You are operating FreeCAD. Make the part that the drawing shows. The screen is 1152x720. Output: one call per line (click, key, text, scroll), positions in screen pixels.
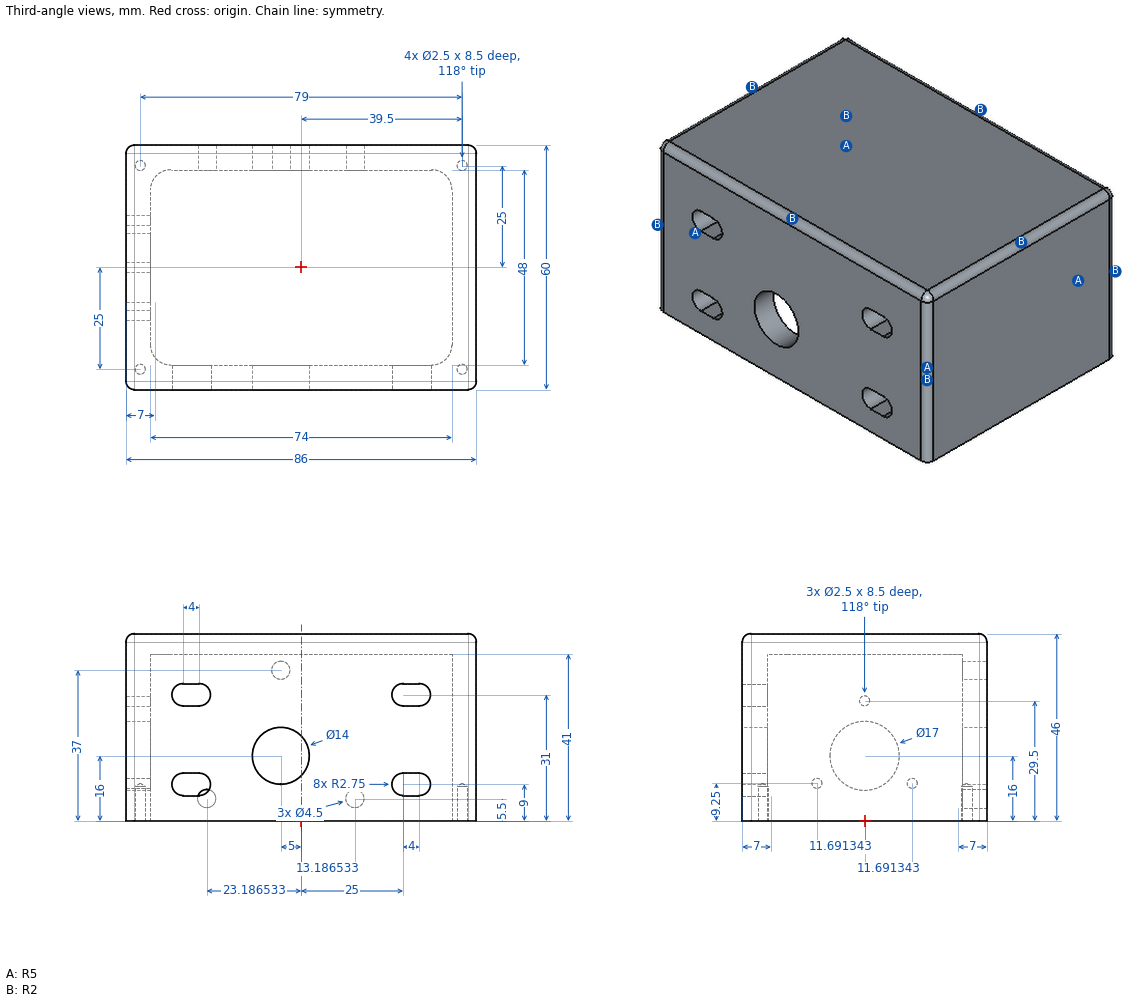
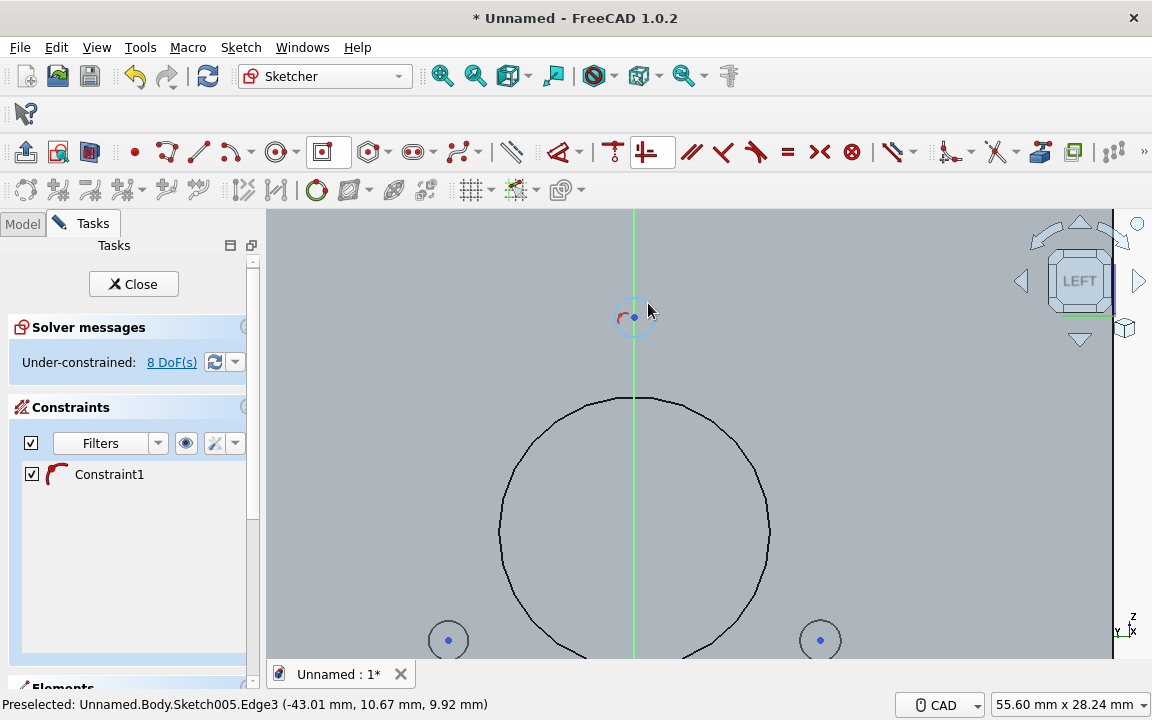
click(648, 304)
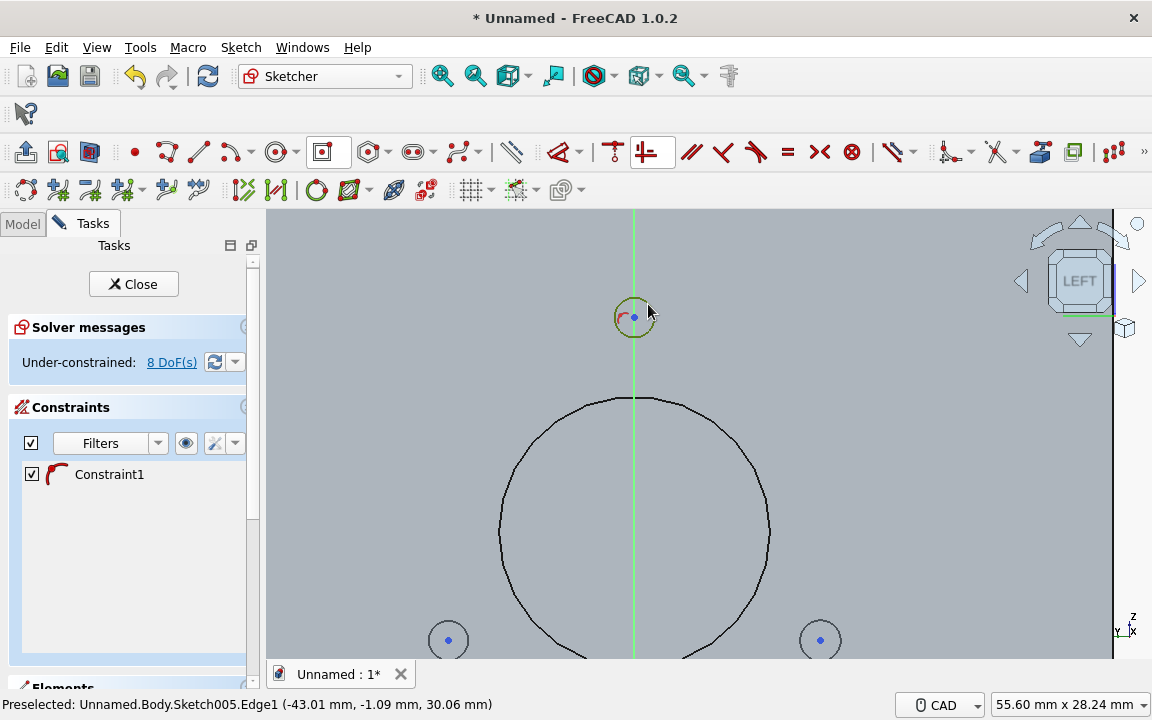
click(835, 626)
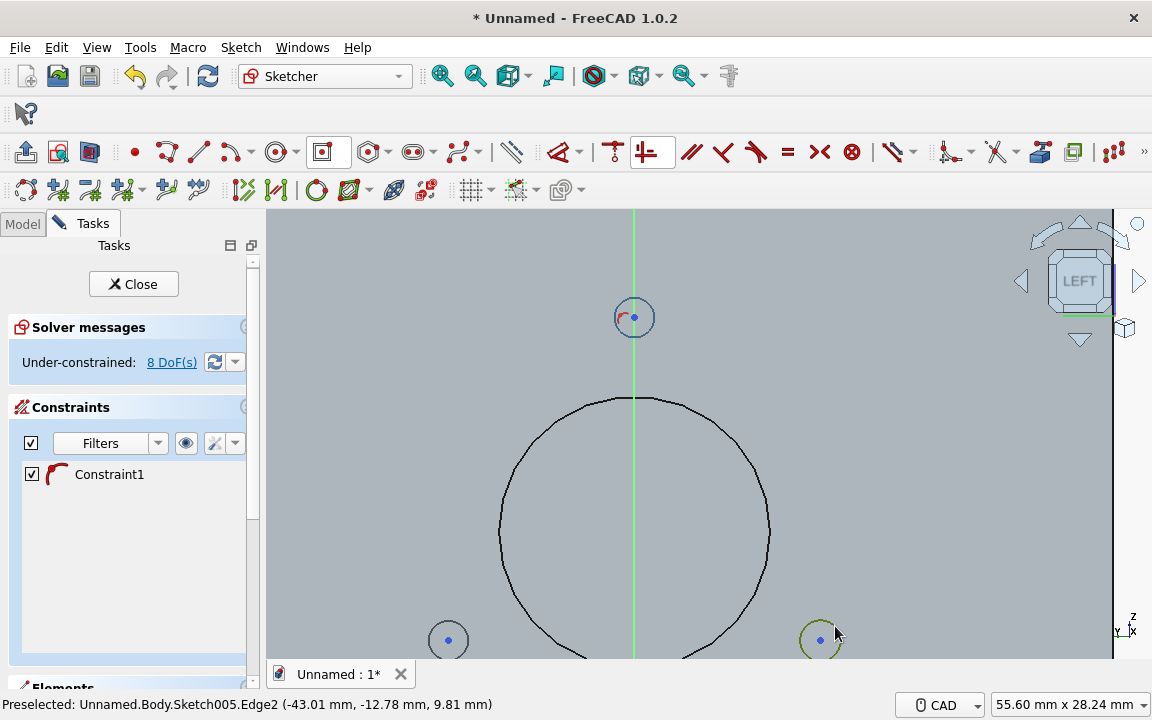
click(462, 627)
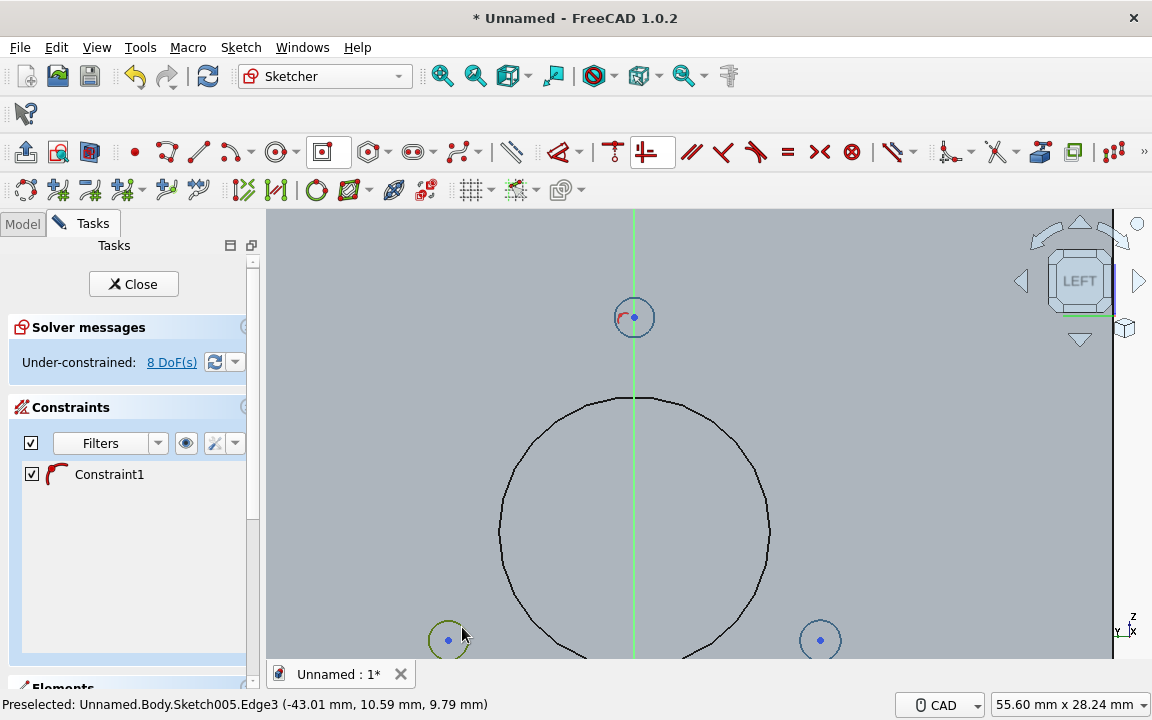
key(e)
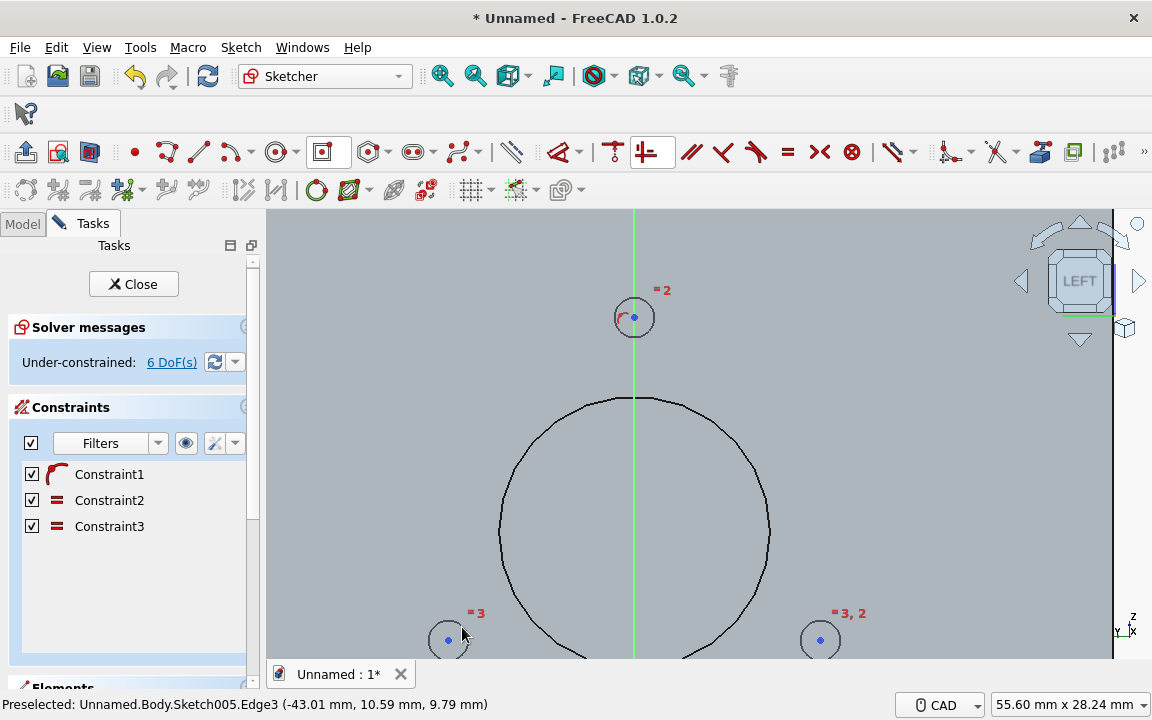
scroll(648, 303, down, 3)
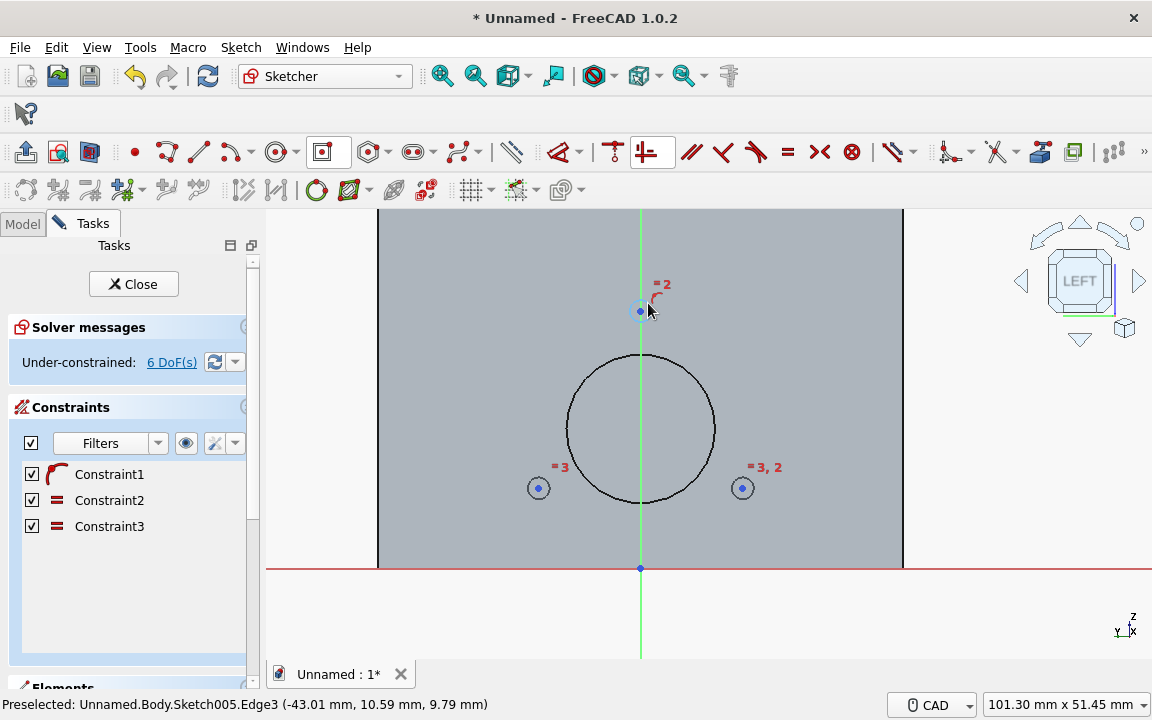
click(743, 488)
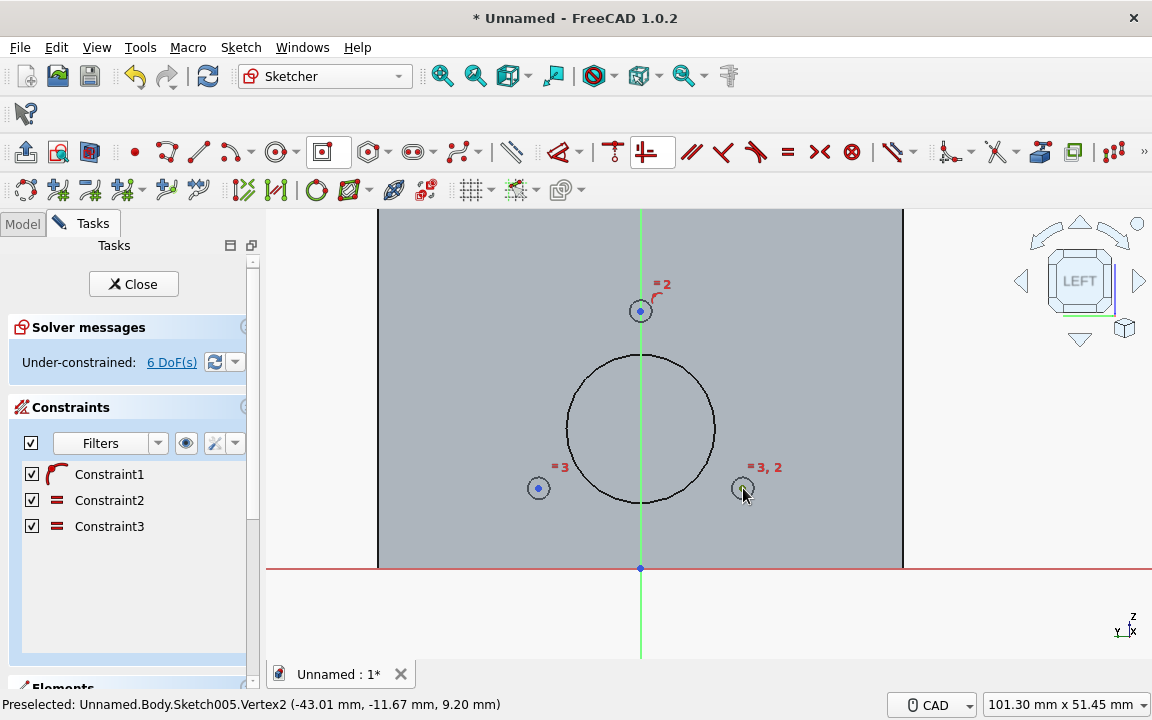
click(539, 488)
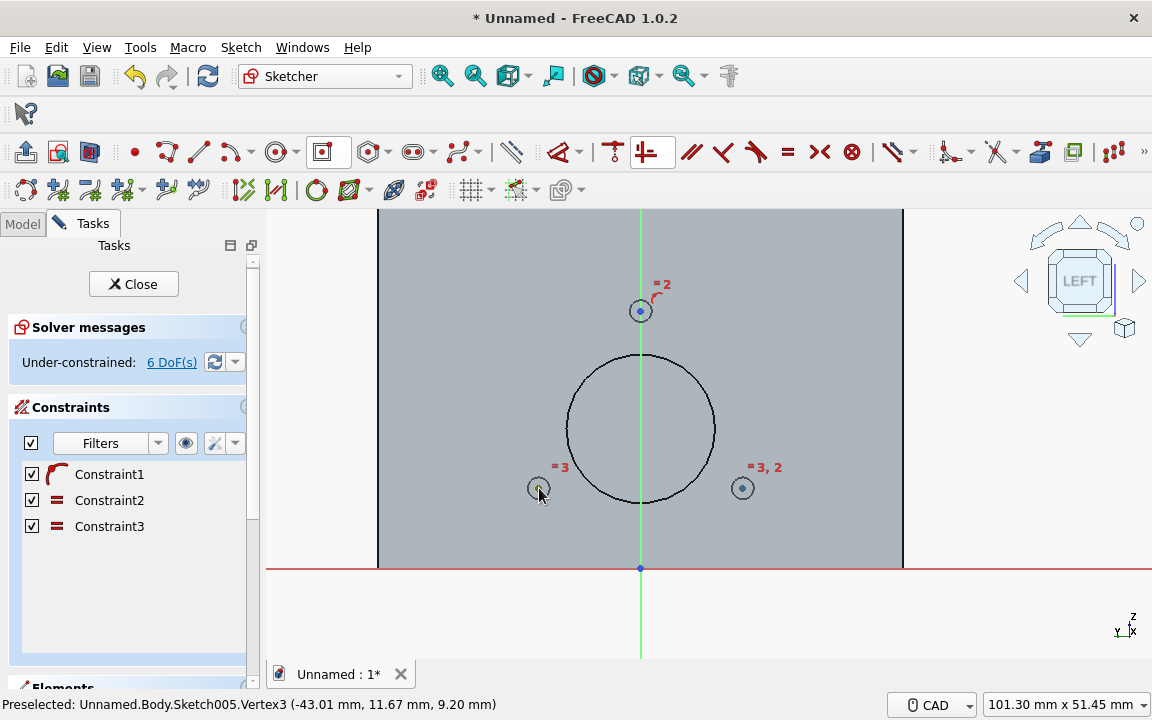
key(h)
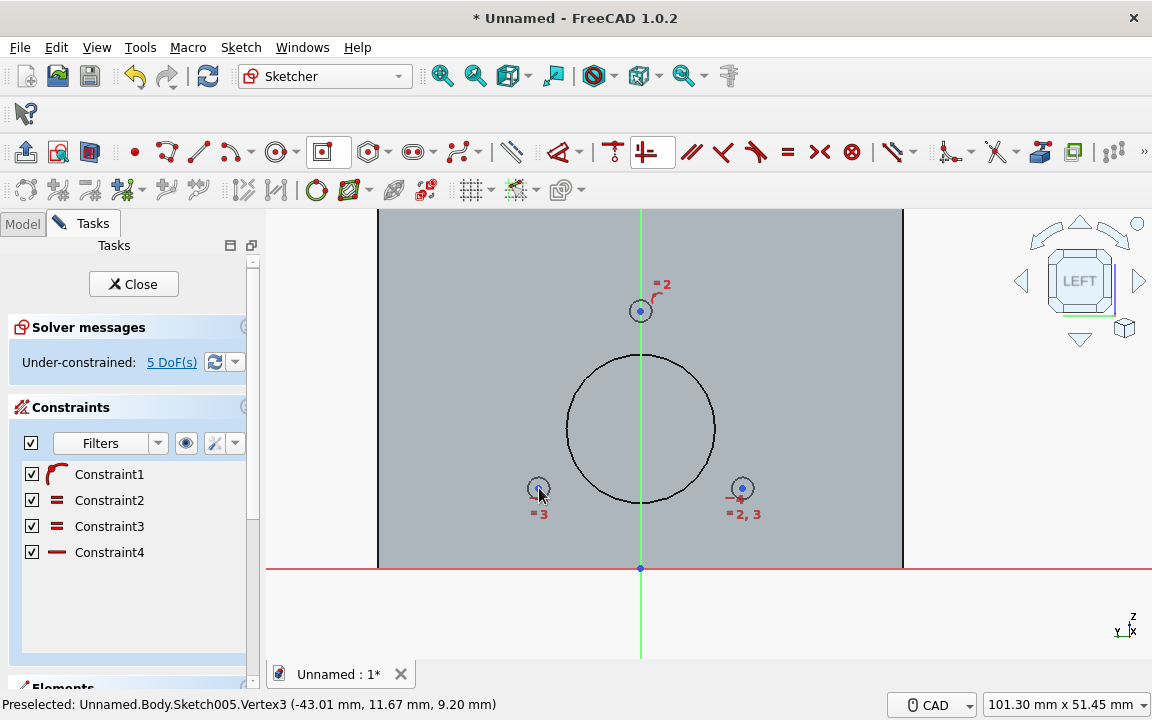
key(d)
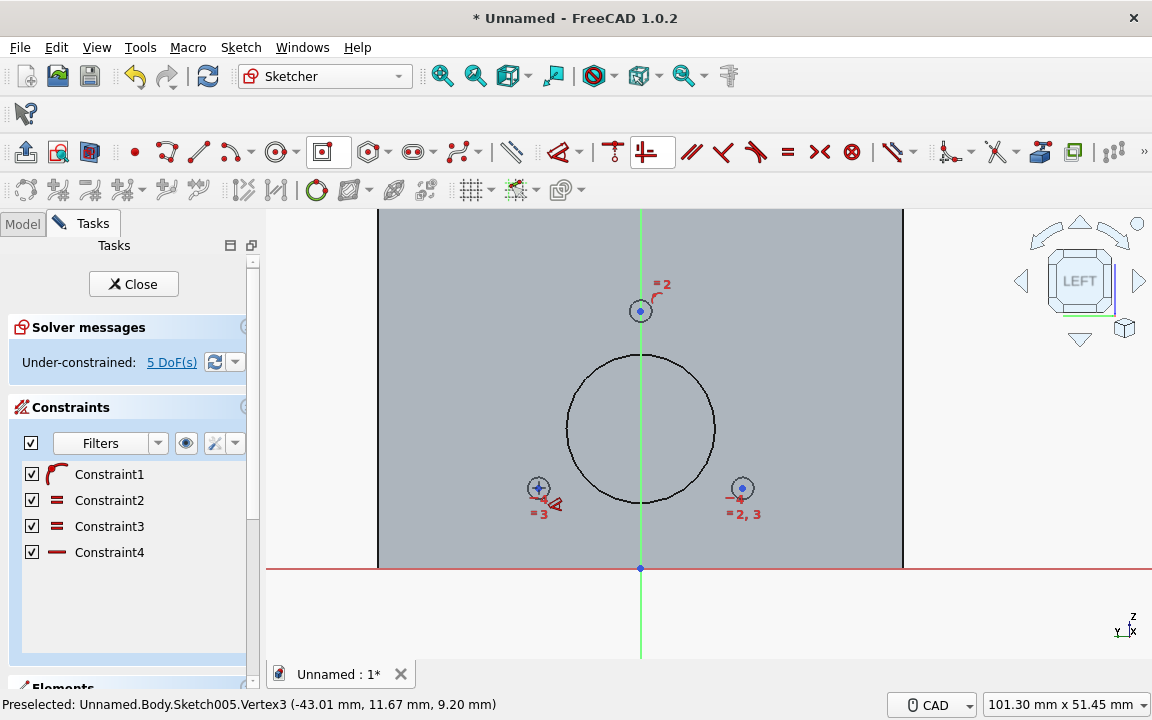
scroll(641, 300, up, 3)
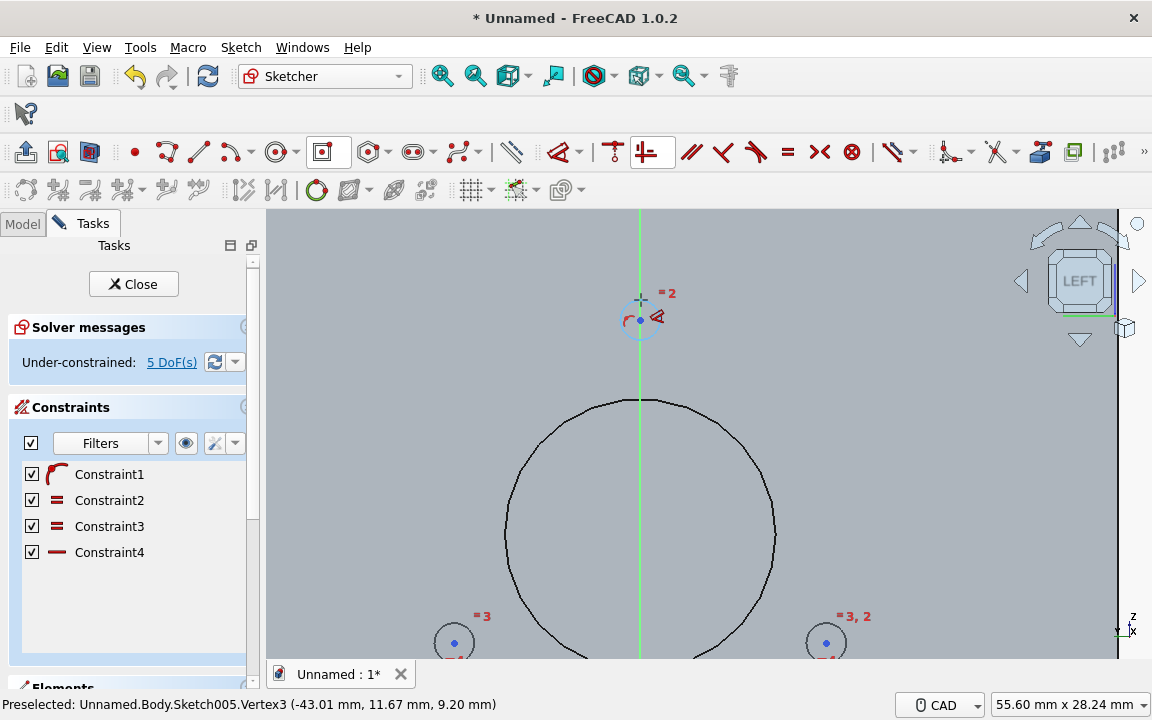
click(641, 300)
click(667, 275)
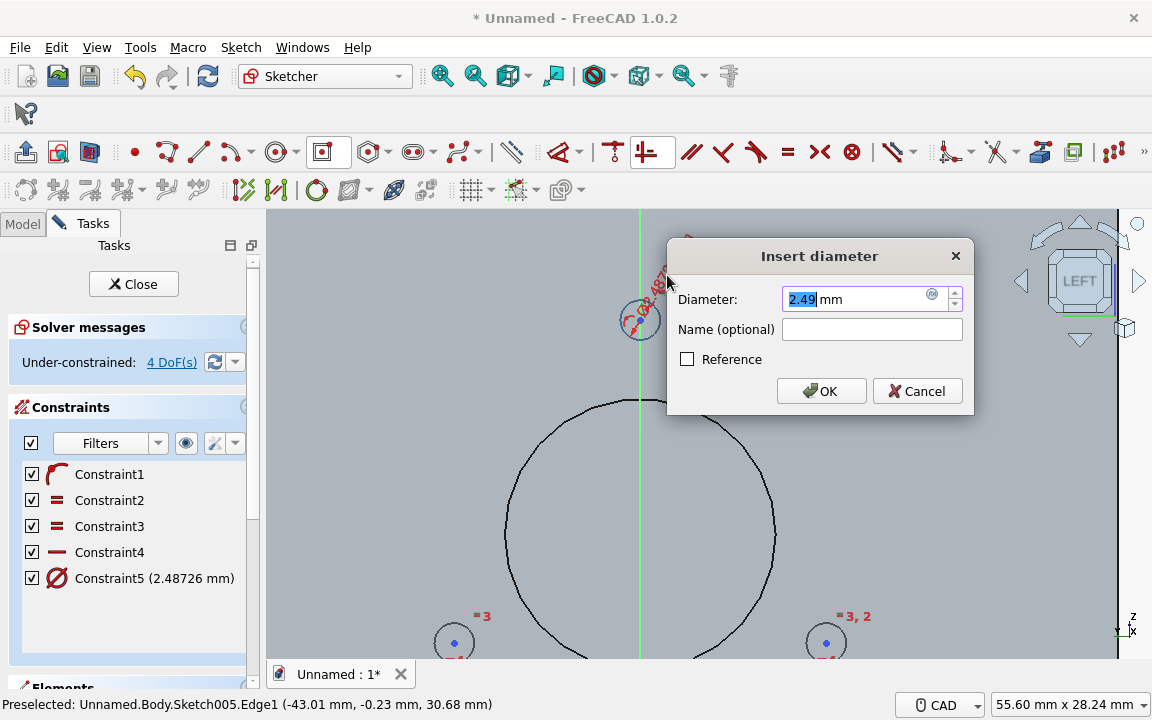
text(2.5)
key(Return)